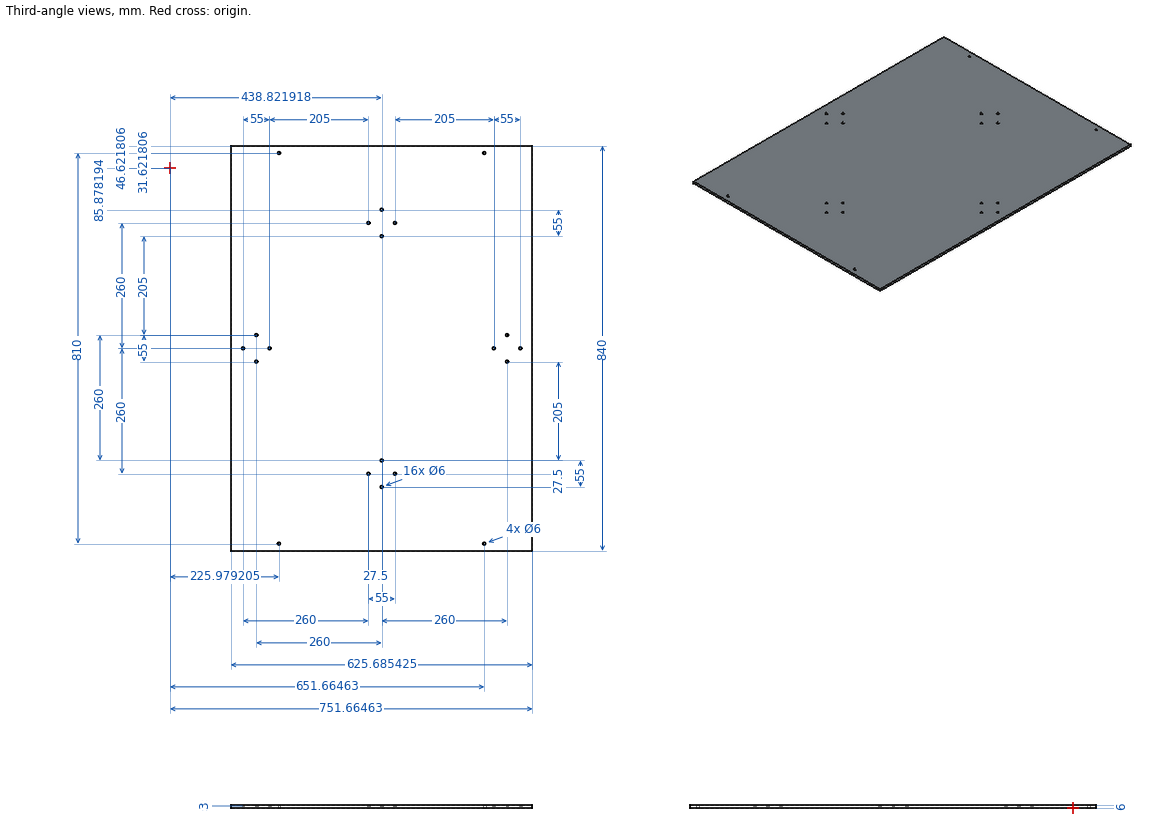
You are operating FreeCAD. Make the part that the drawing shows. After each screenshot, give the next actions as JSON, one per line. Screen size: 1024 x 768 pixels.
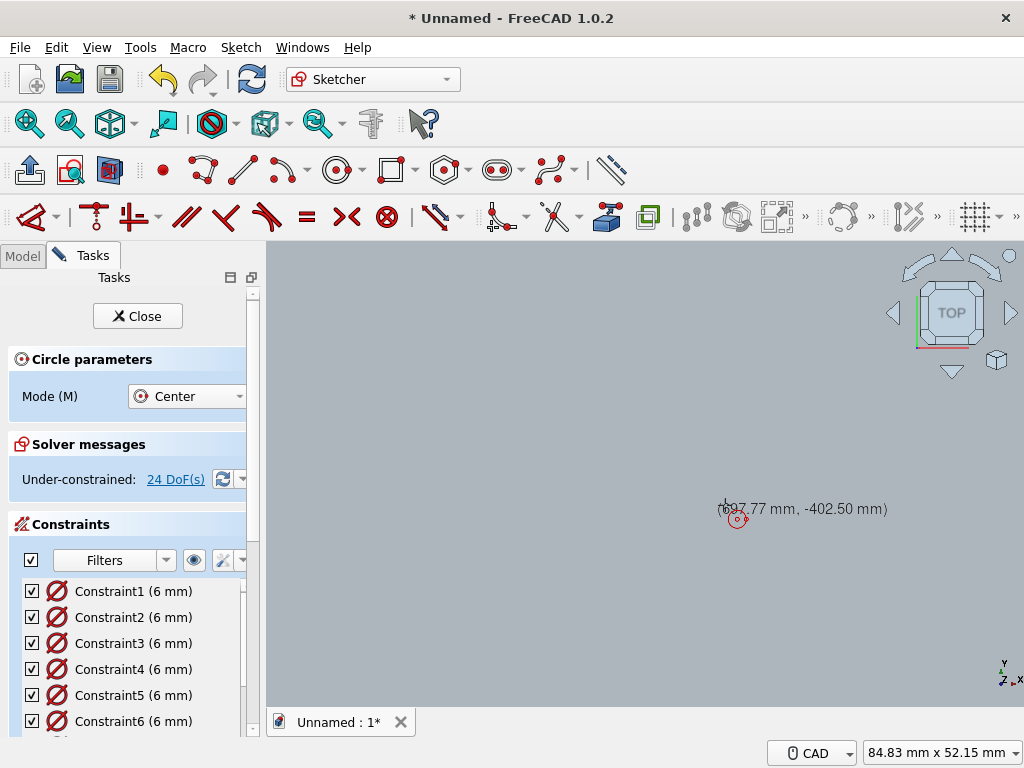
{"action": "scroll", "coordinate": [725, 505], "scroll_direction": "down", "scroll_amount": 15}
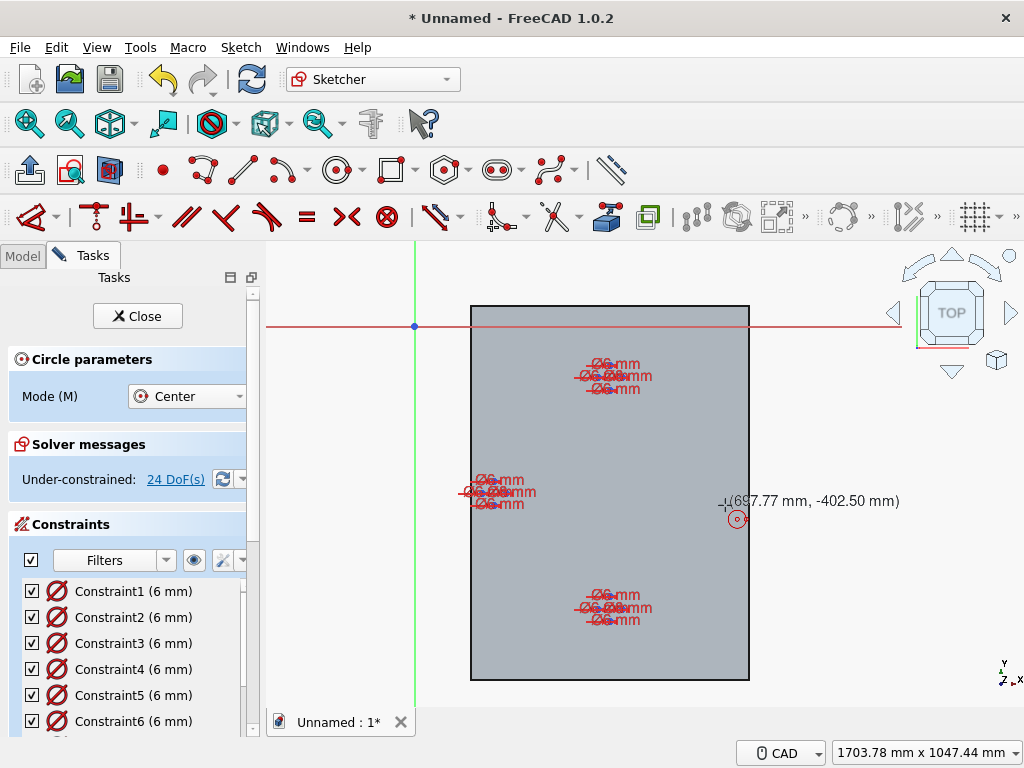
{"action": "left_click", "coordinate": [725, 505]}
{"action": "mouse_move", "coordinate": [726, 504]}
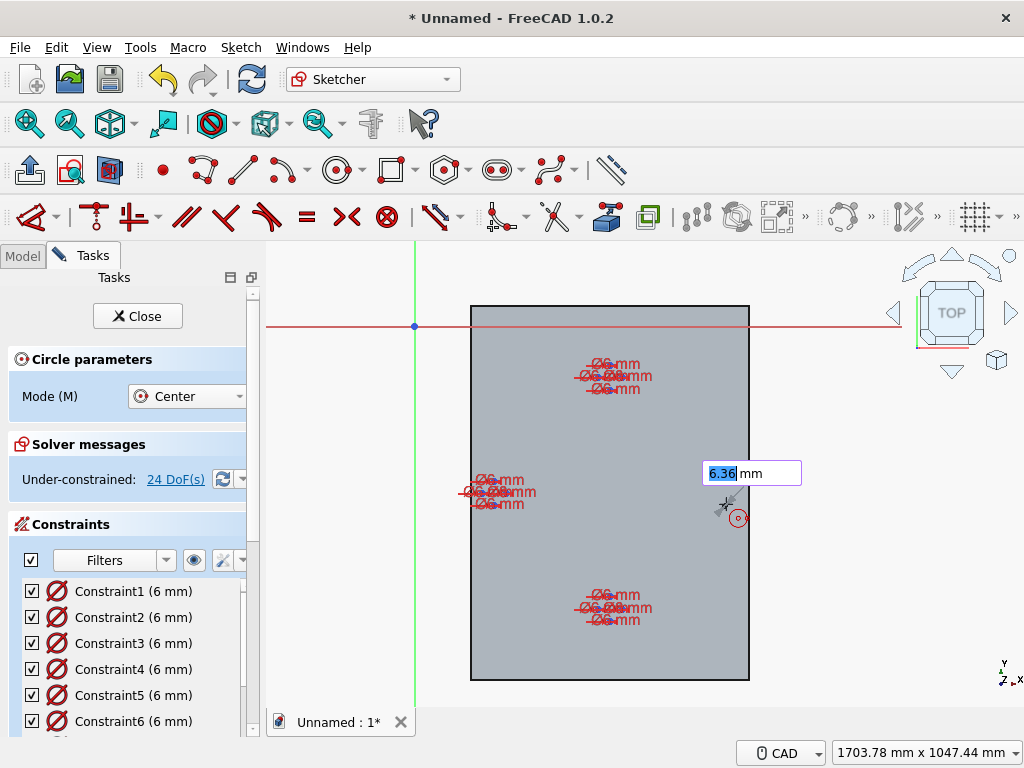
{"action": "type", "text": "6"}
{"action": "key", "text": "Return"}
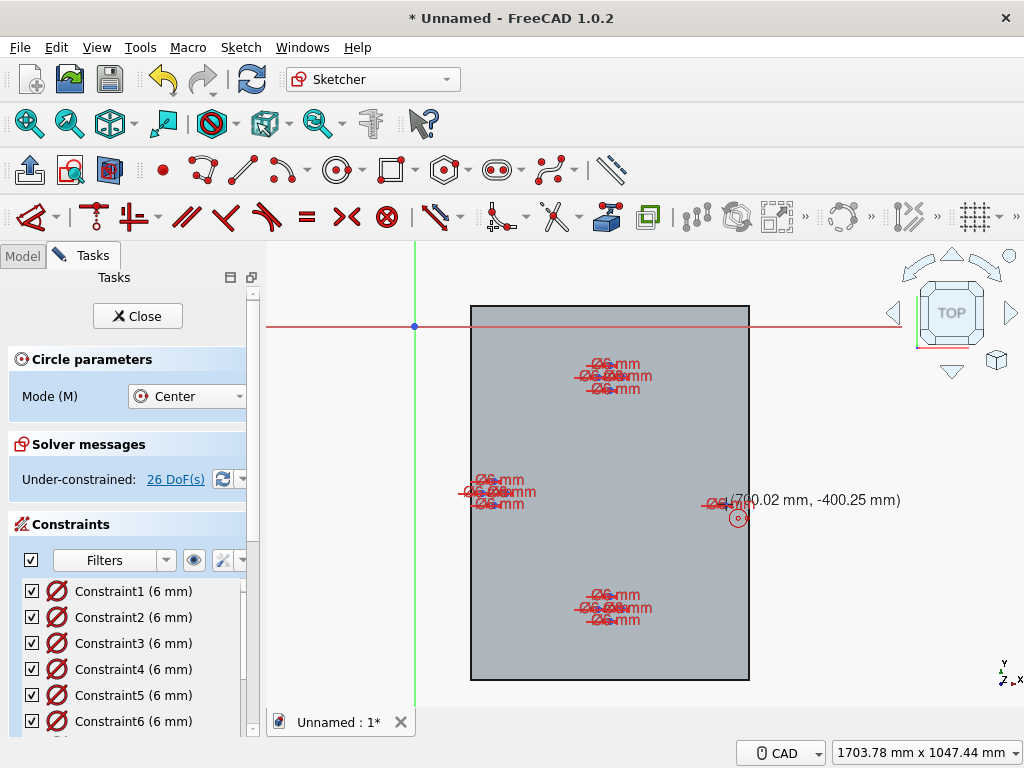
{"action": "scroll", "coordinate": [713, 493], "scroll_direction": "up", "scroll_amount": 15}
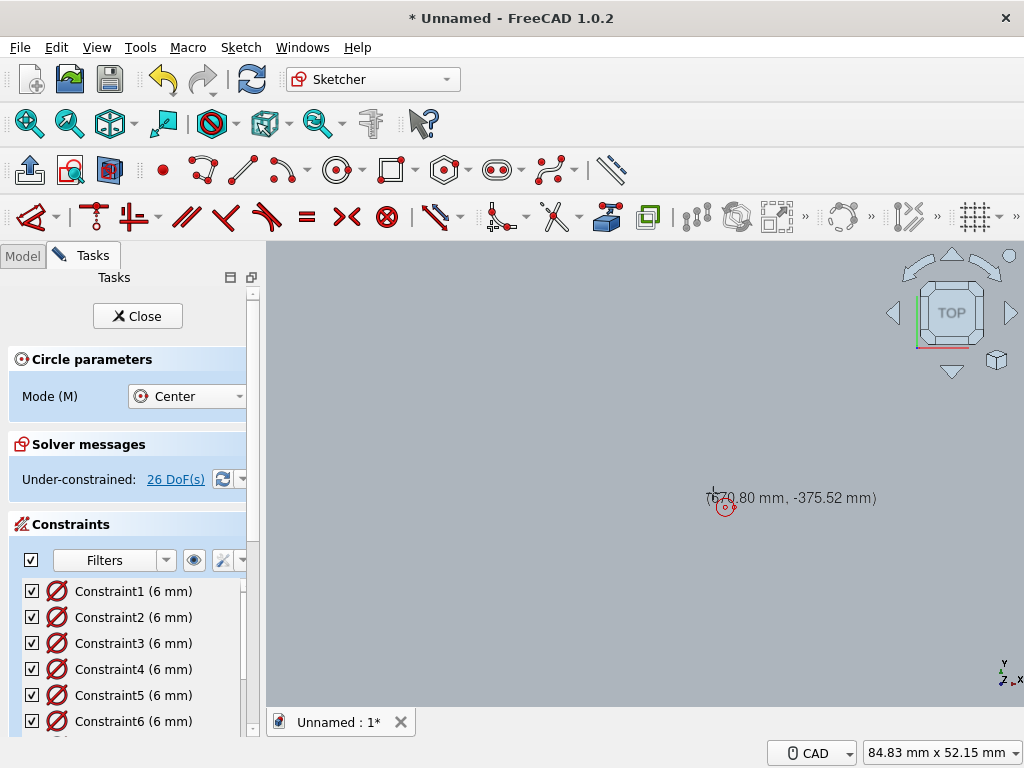
{"action": "scroll", "coordinate": [713, 493], "scroll_direction": "down", "scroll_amount": 15}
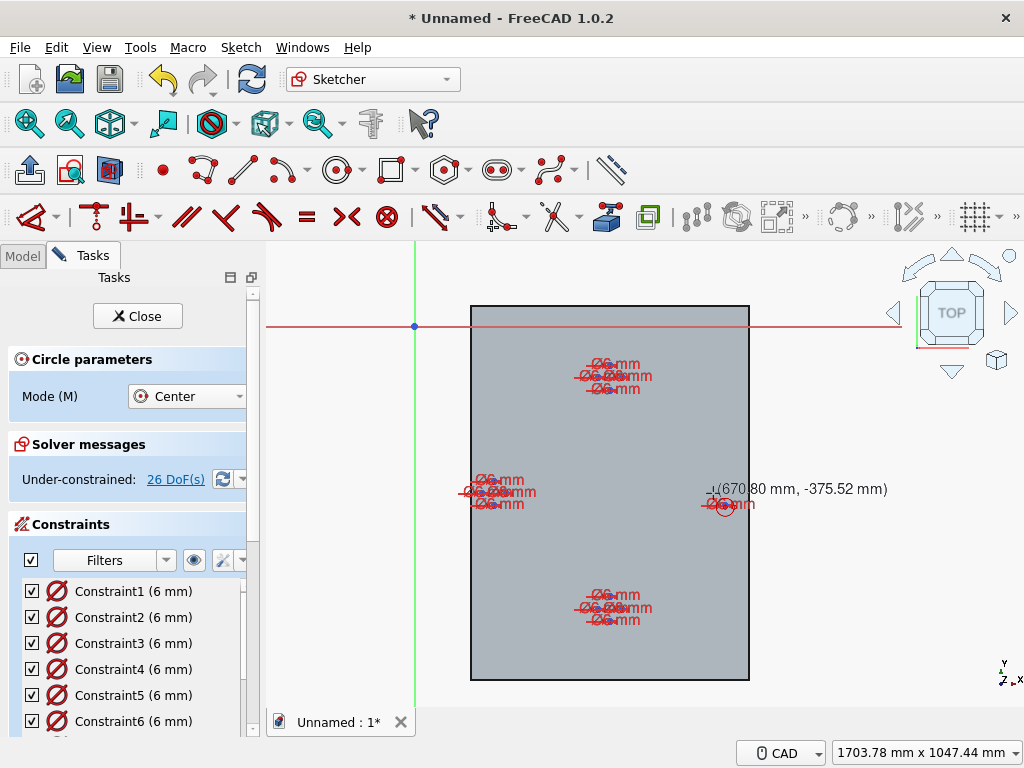
{"action": "left_click", "coordinate": [713, 493]}
{"action": "mouse_move", "coordinate": [714, 492]}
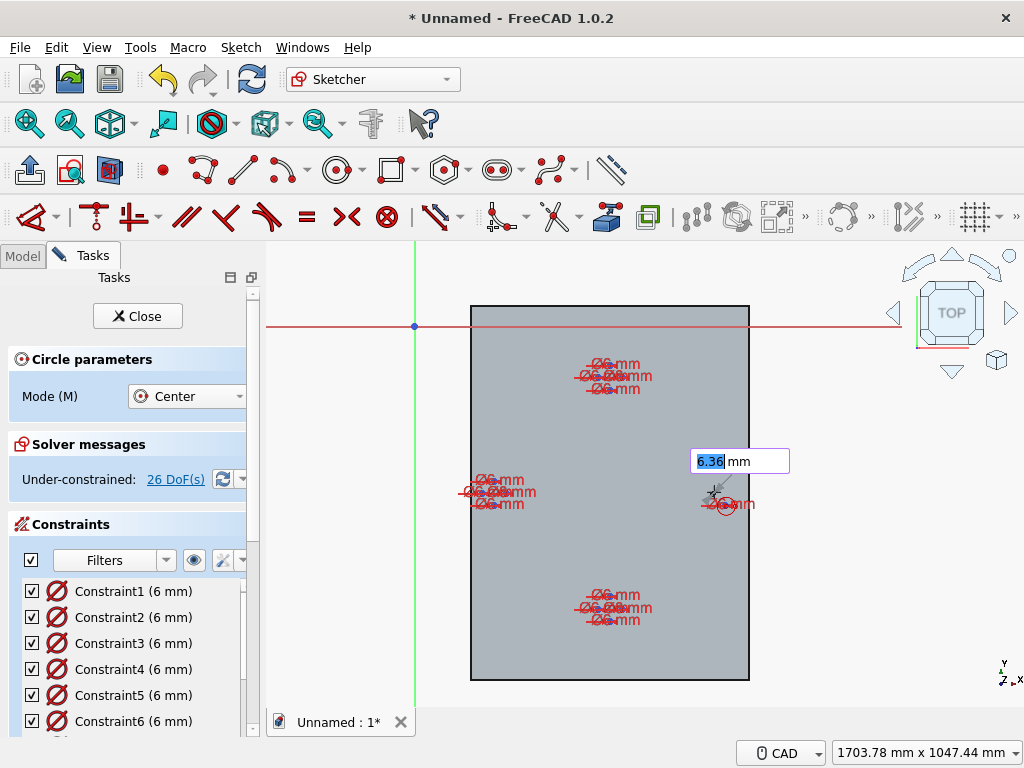
{"action": "type", "text": "6"}
{"action": "key", "text": "Return"}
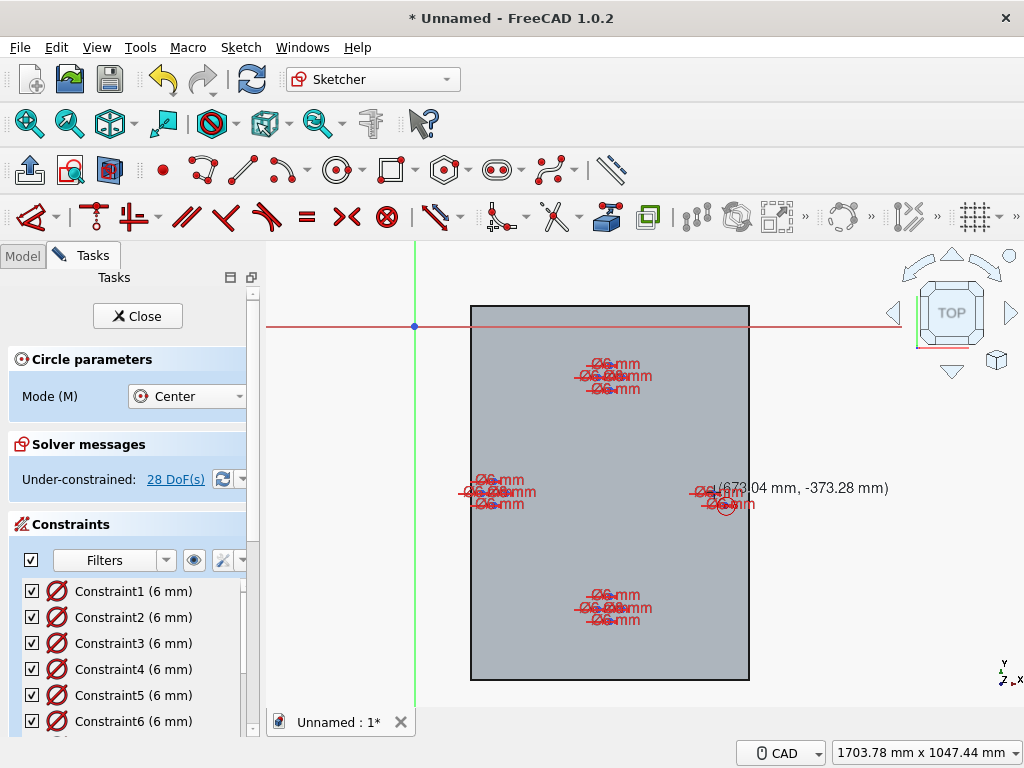
{"action": "scroll", "coordinate": [725, 481], "scroll_direction": "up", "scroll_amount": 15}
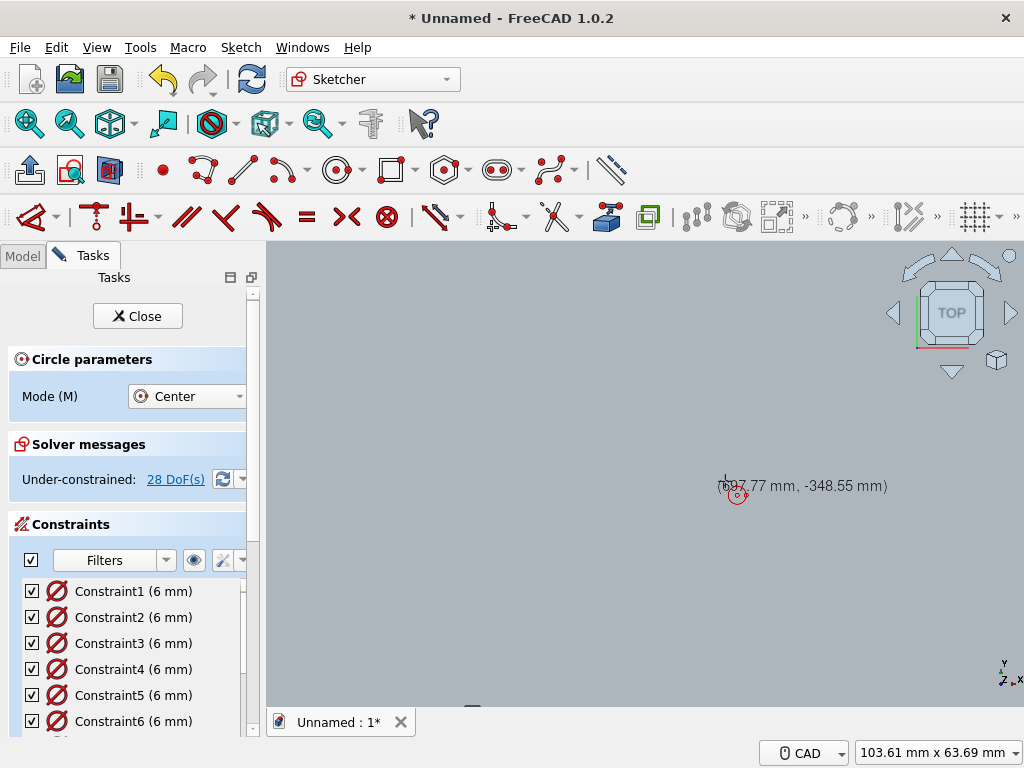
{"action": "scroll", "coordinate": [725, 481], "scroll_direction": "down", "scroll_amount": 15}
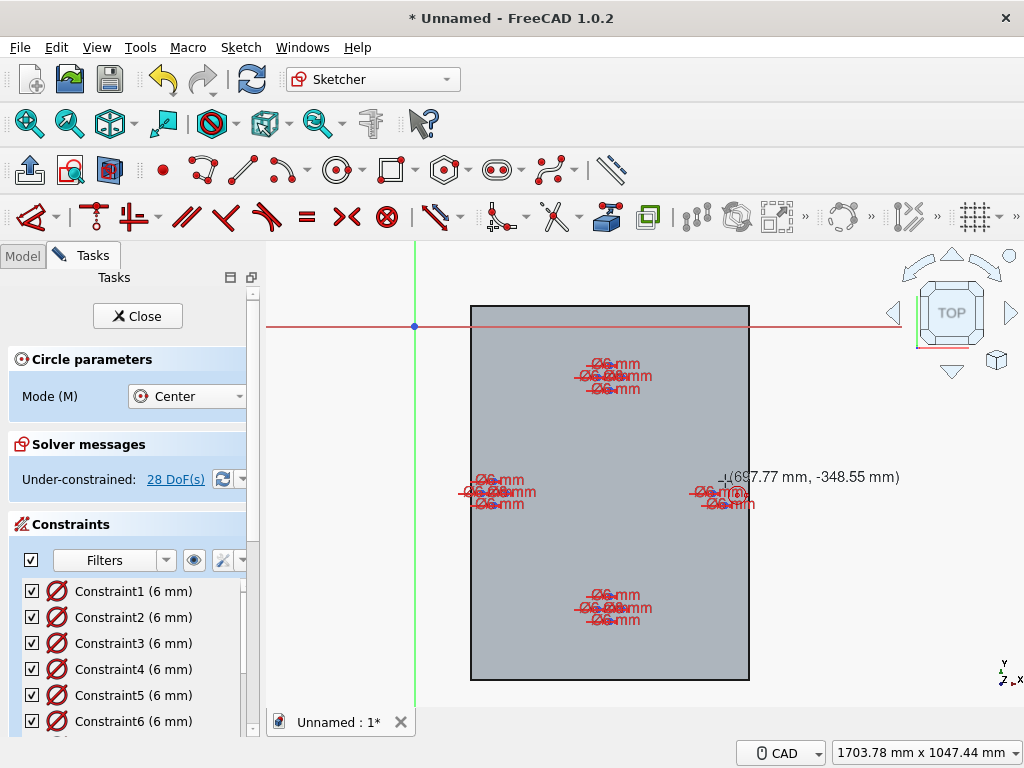
{"action": "left_click", "coordinate": [725, 481]}
{"action": "mouse_move", "coordinate": [726, 480]}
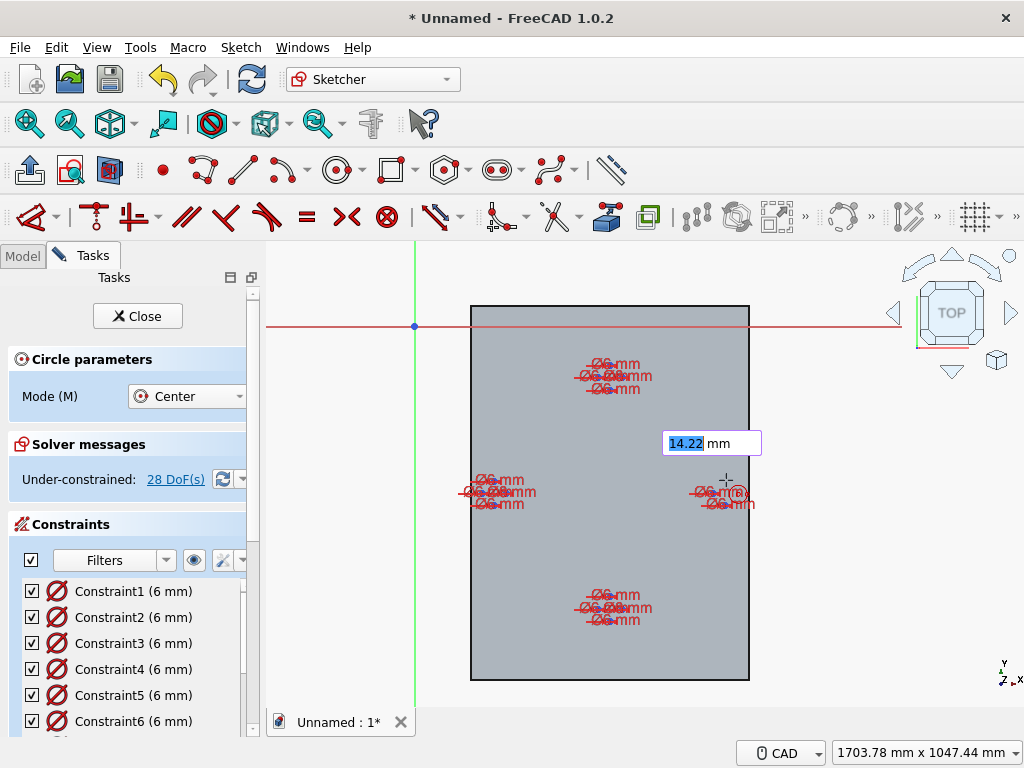
{"action": "type", "text": "6"}
{"action": "key", "text": "Return"}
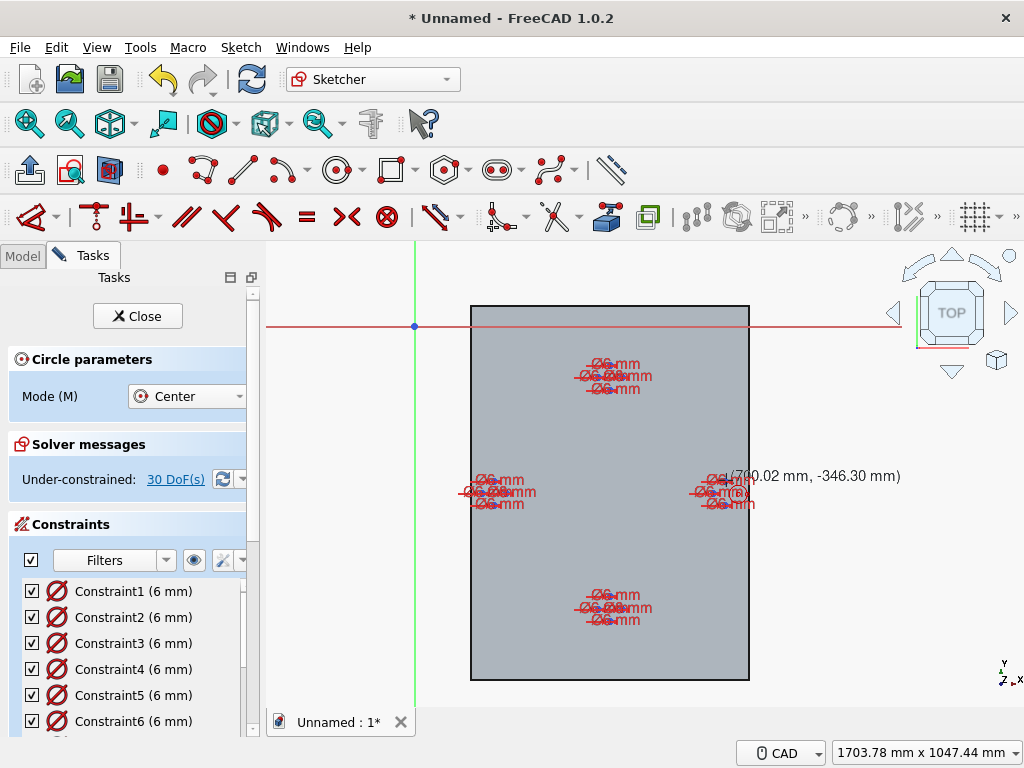
{"action": "scroll", "coordinate": [738, 493], "scroll_direction": "up", "scroll_amount": 15}